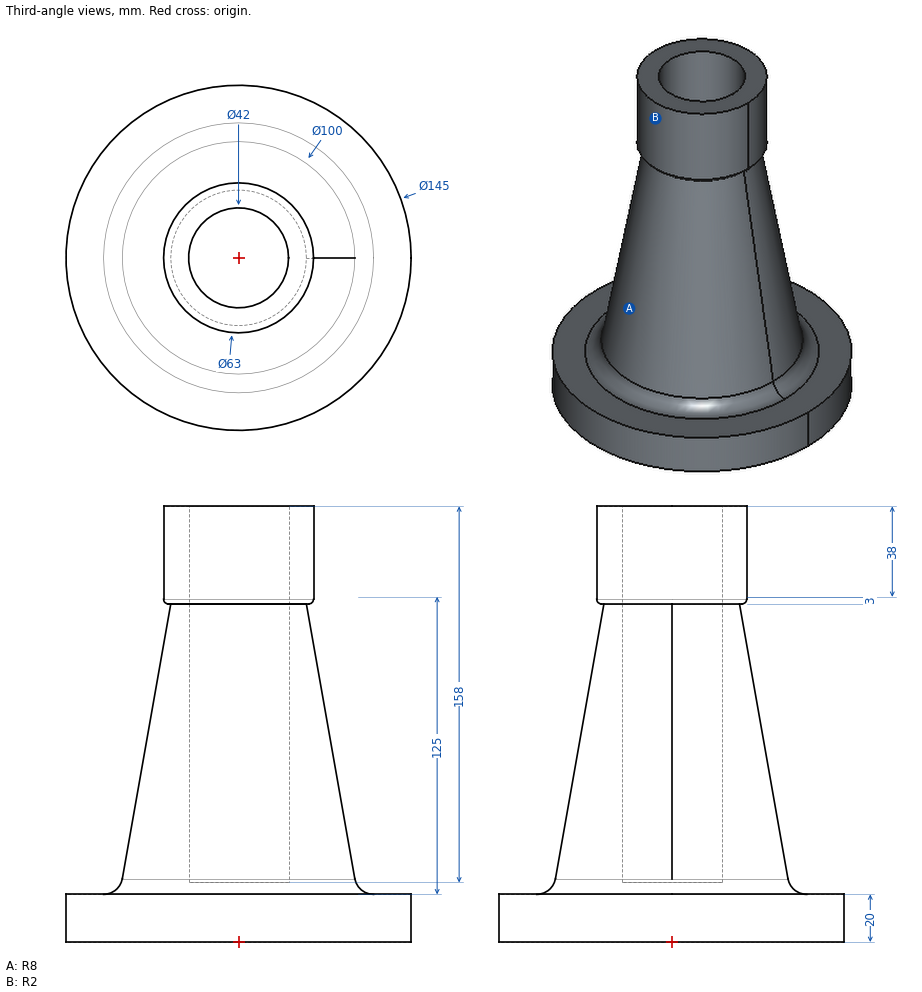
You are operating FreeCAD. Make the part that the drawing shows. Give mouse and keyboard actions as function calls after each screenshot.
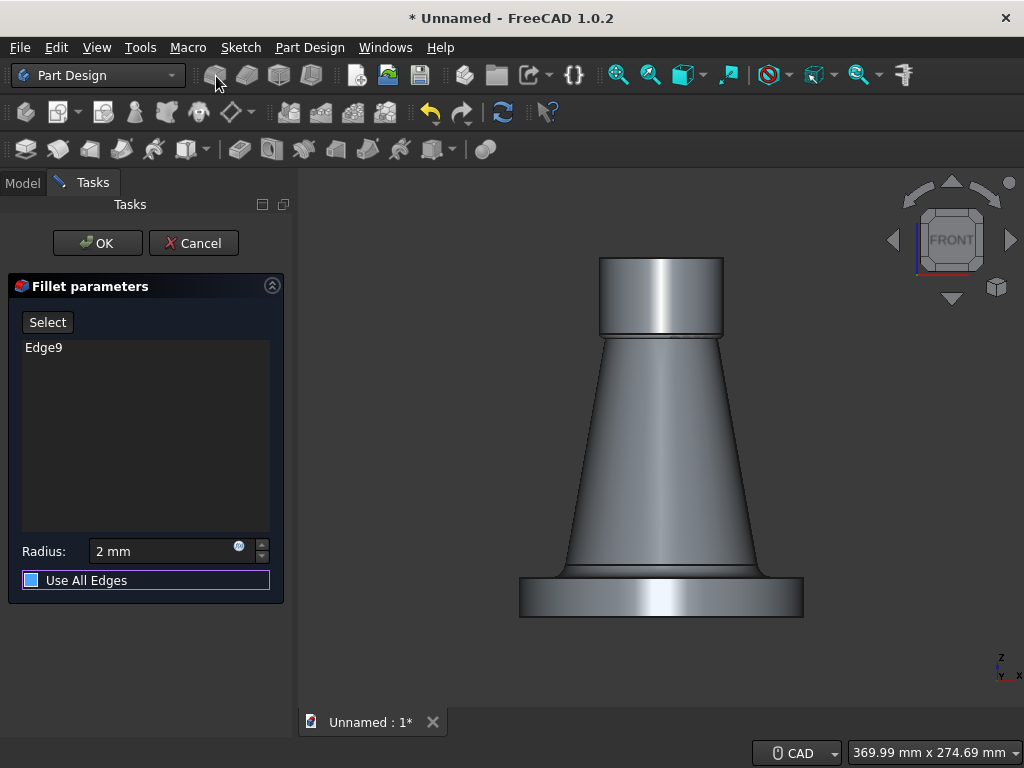
click(98, 243)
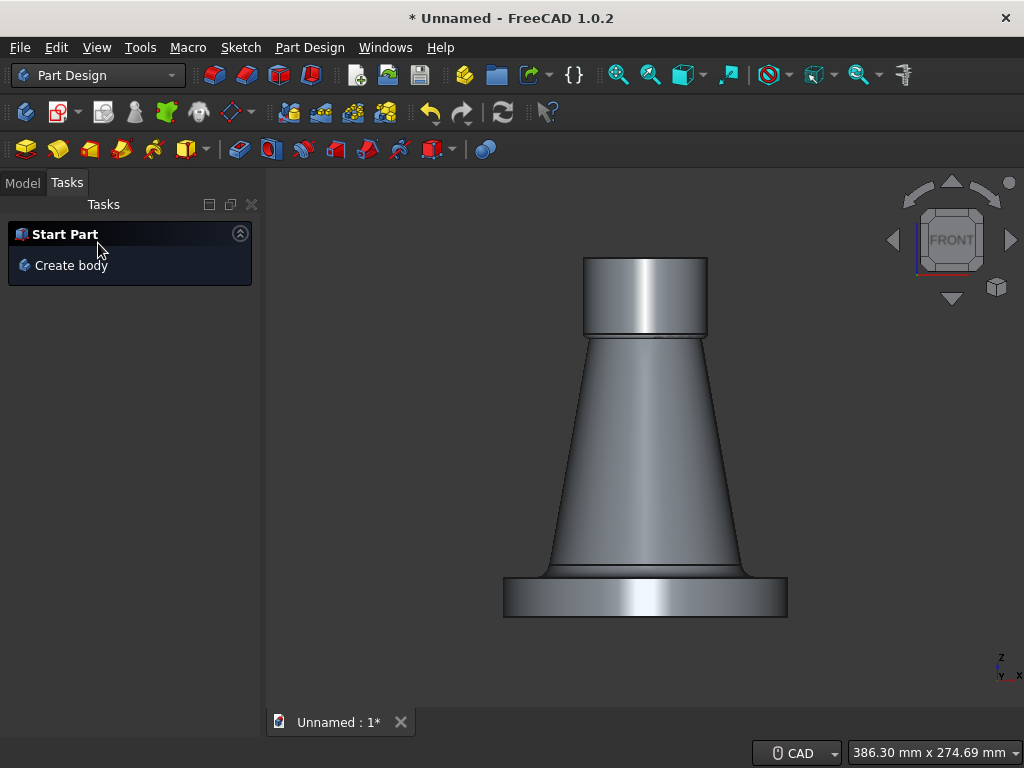
key(0)